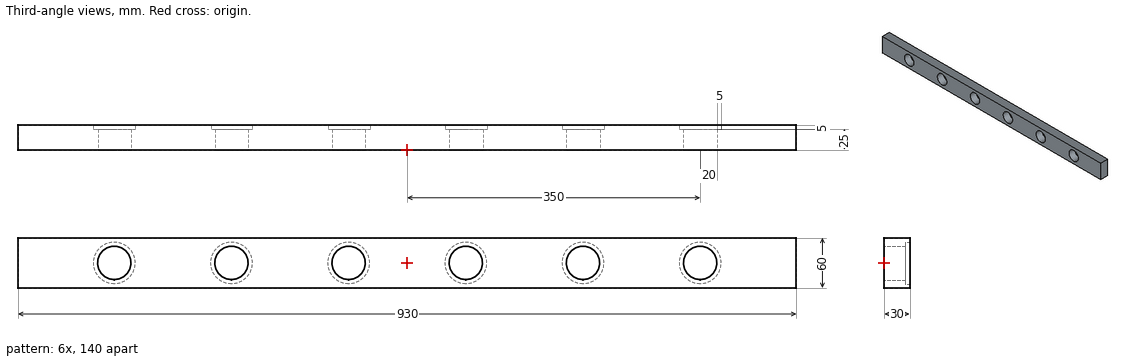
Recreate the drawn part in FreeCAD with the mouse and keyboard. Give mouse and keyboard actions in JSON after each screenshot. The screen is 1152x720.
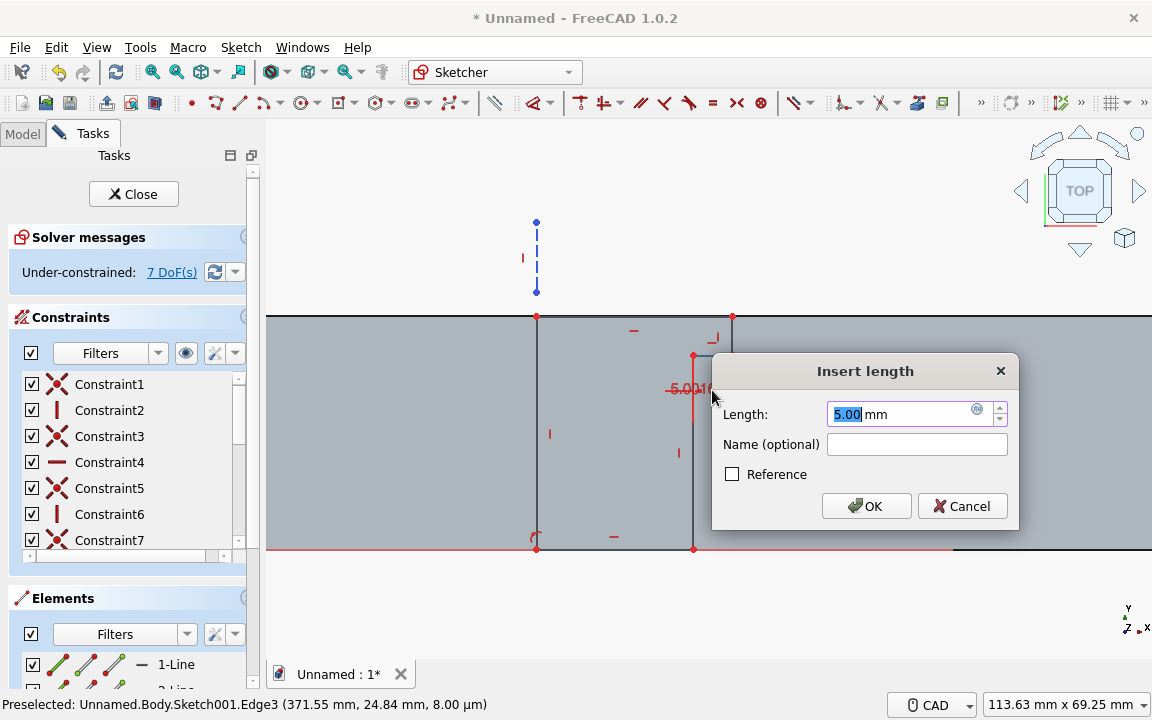
{"action": "type", "text": "5"}
{"action": "key", "text": "Return"}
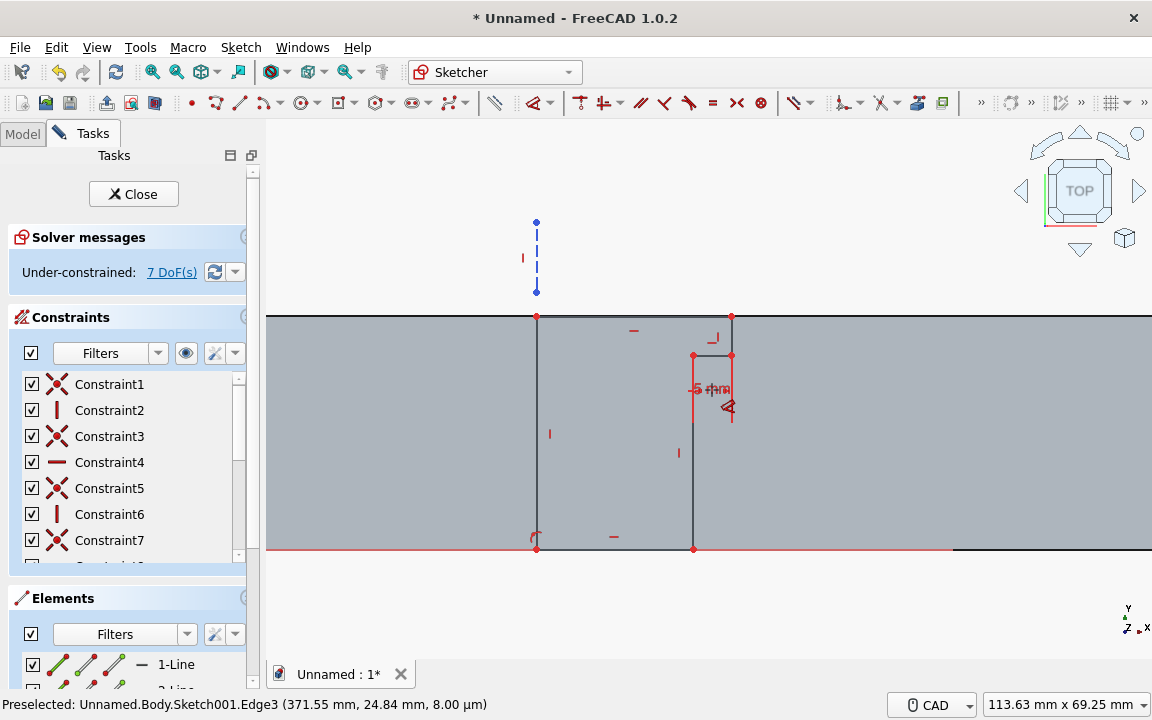
{"action": "left_click", "coordinate": [732, 344]}
{"action": "left_click", "coordinate": [766, 337]}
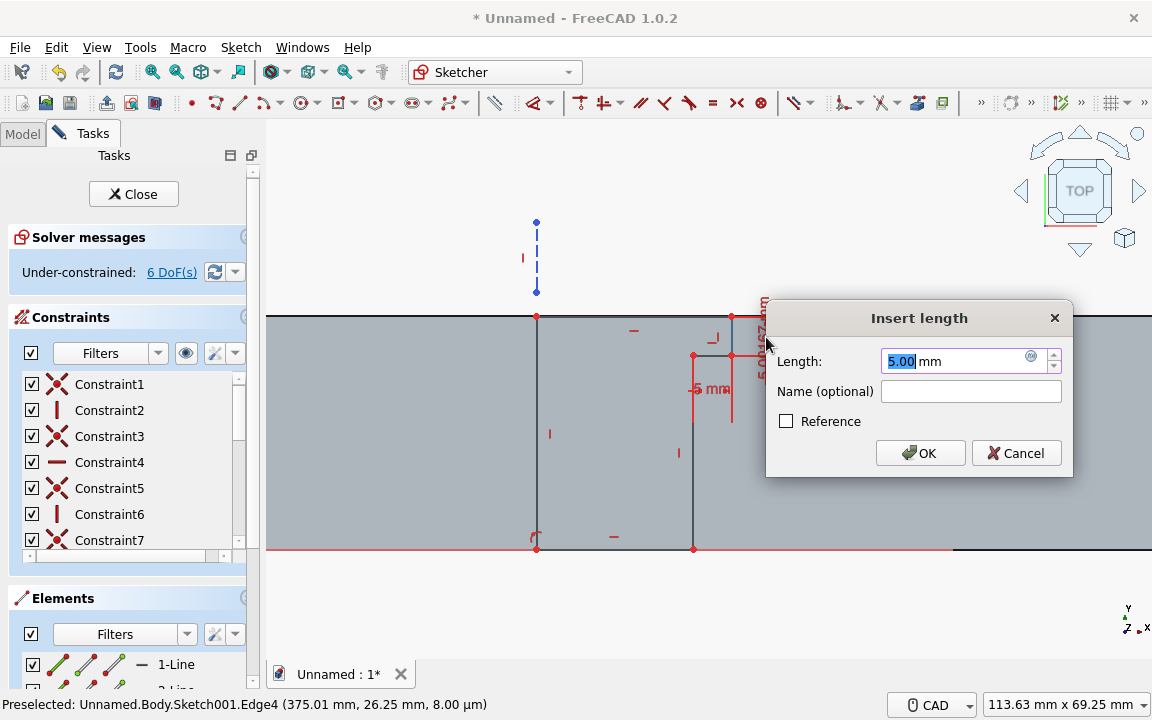
{"action": "type", "text": "5"}
{"action": "key", "text": "Return"}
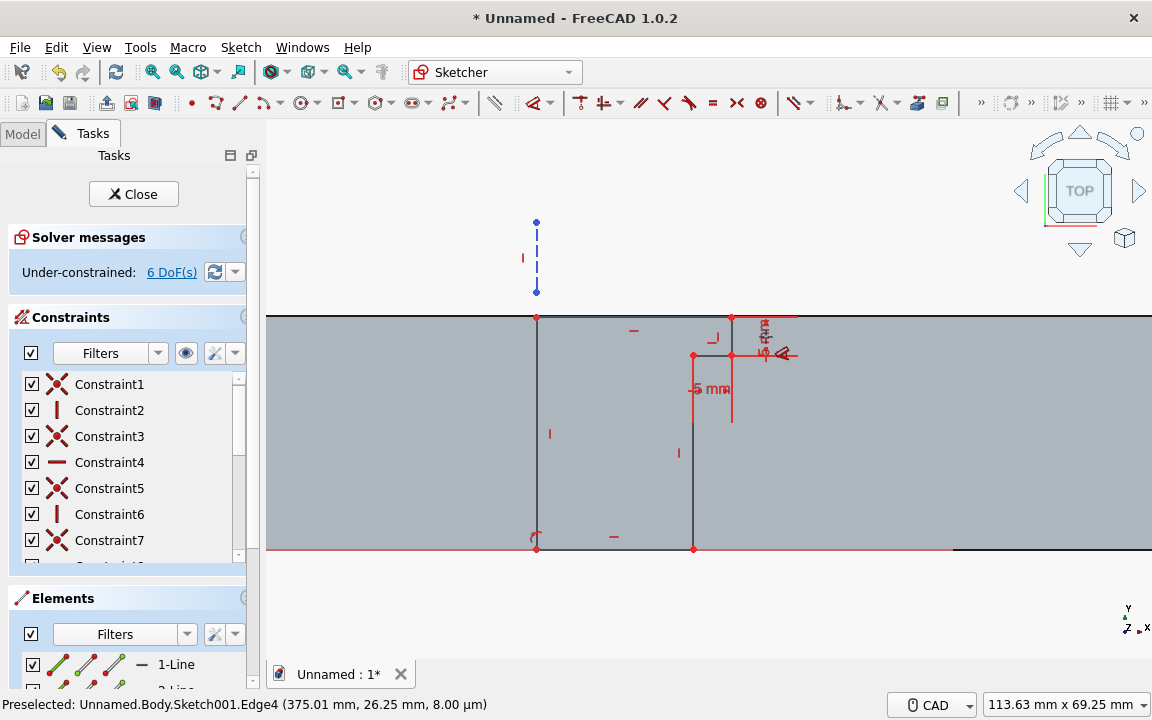
{"action": "left_click", "coordinate": [584, 550]}
{"action": "left_click", "coordinate": [615, 584]}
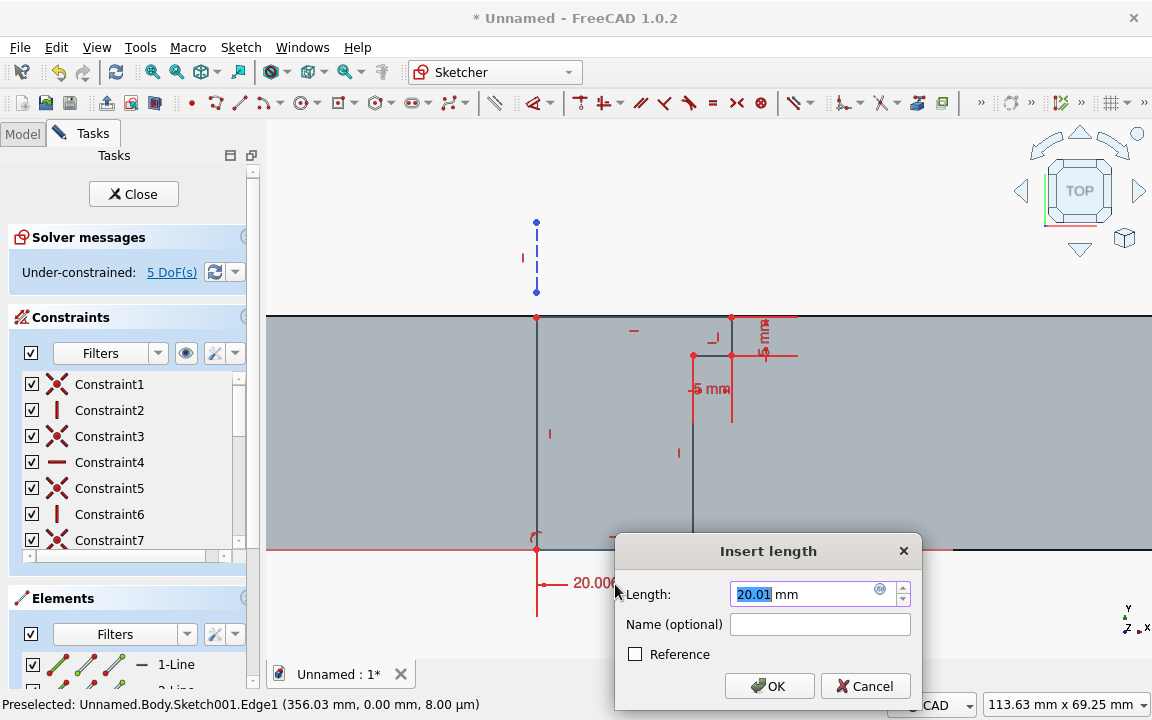
{"action": "type", "text": "20"}
{"action": "key", "text": "Return"}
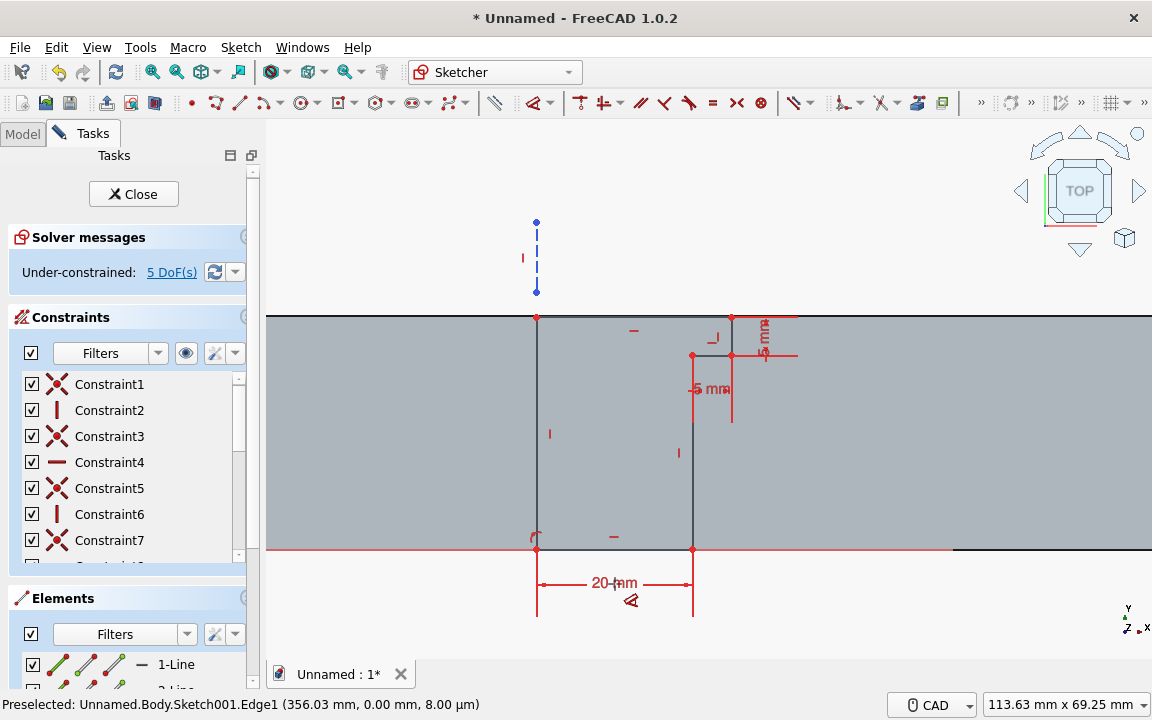
{"action": "left_click", "coordinate": [693, 492]}
{"action": "left_click", "coordinate": [727, 453]}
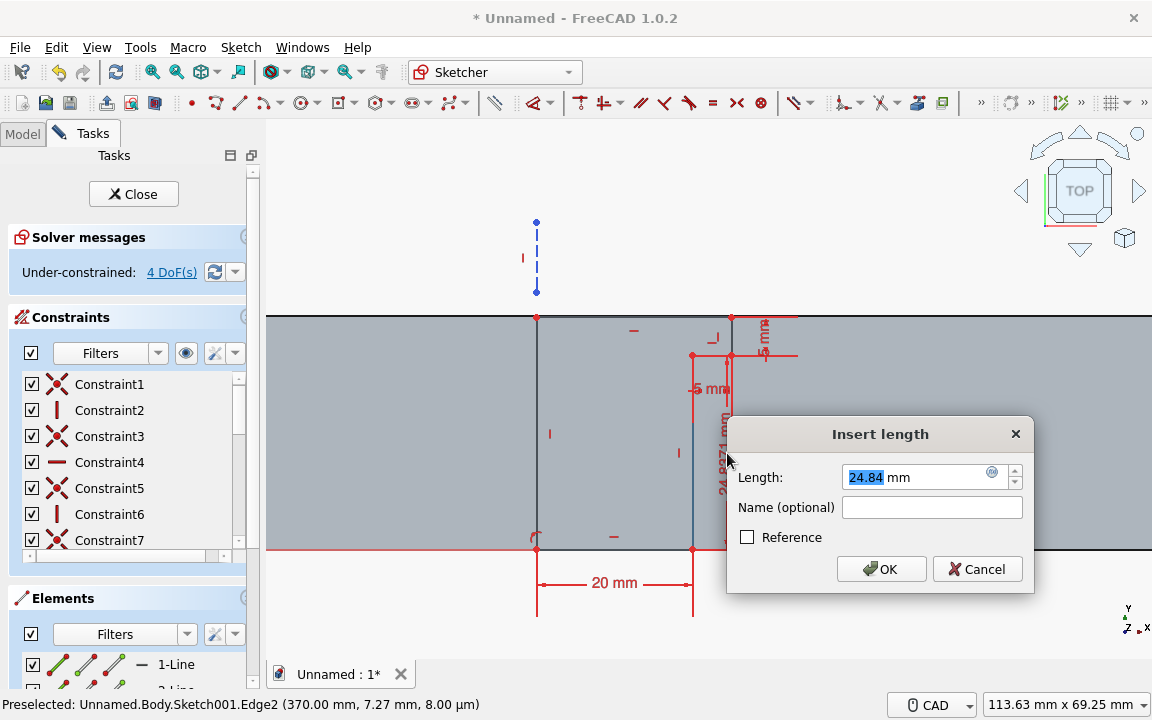
{"action": "type", "text": "25"}
{"action": "key", "text": "Return"}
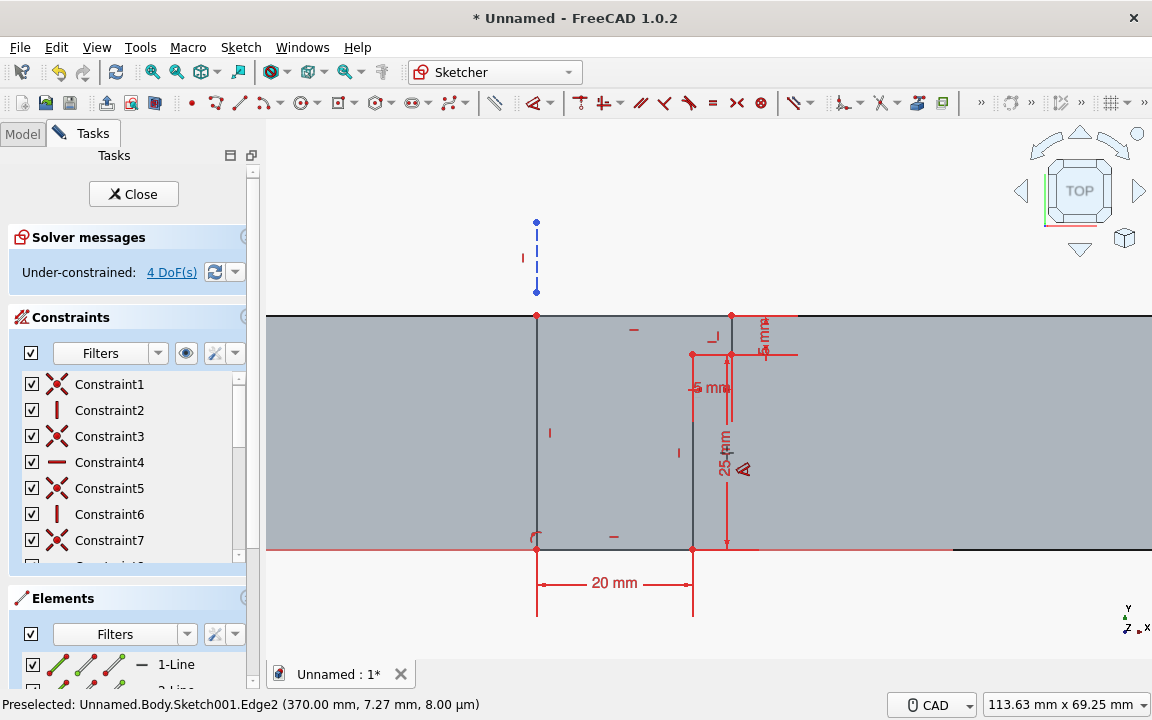
{"action": "left_click", "coordinate": [537, 550]}
{"action": "left_click", "coordinate": [415, 584]}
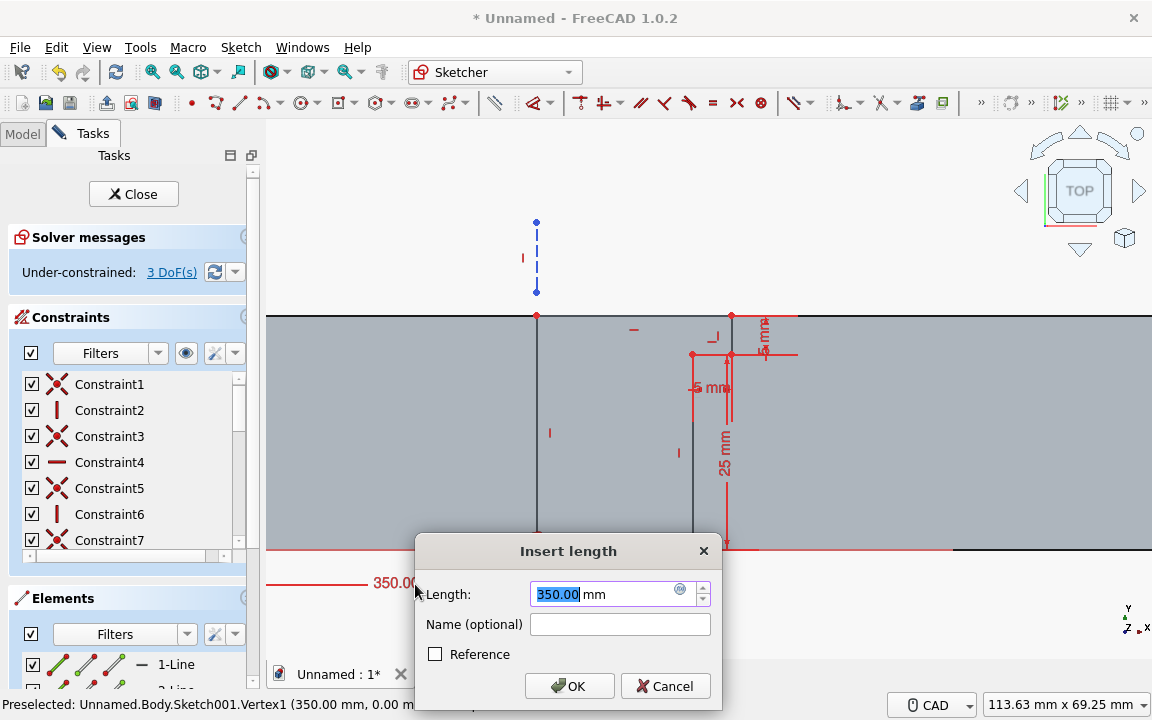
{"action": "type", "text": "350"}
{"action": "key", "text": "Return"}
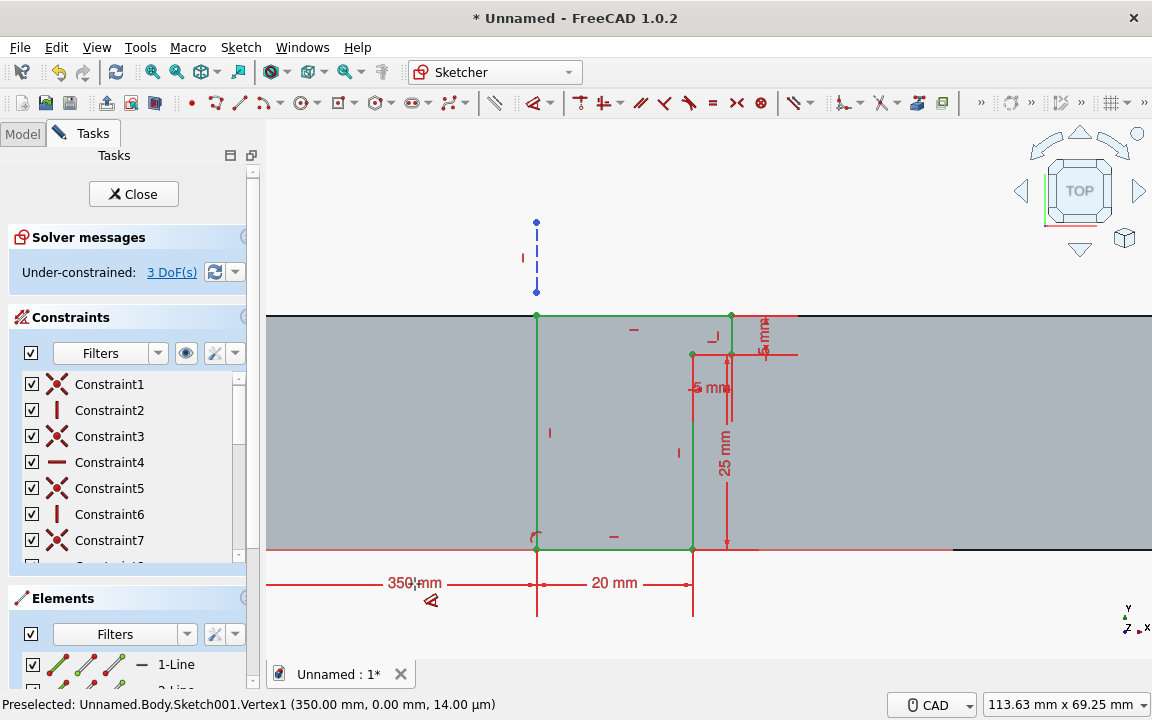
{"action": "left_click", "coordinate": [537, 293]}
{"action": "left_click", "coordinate": [330, 584]}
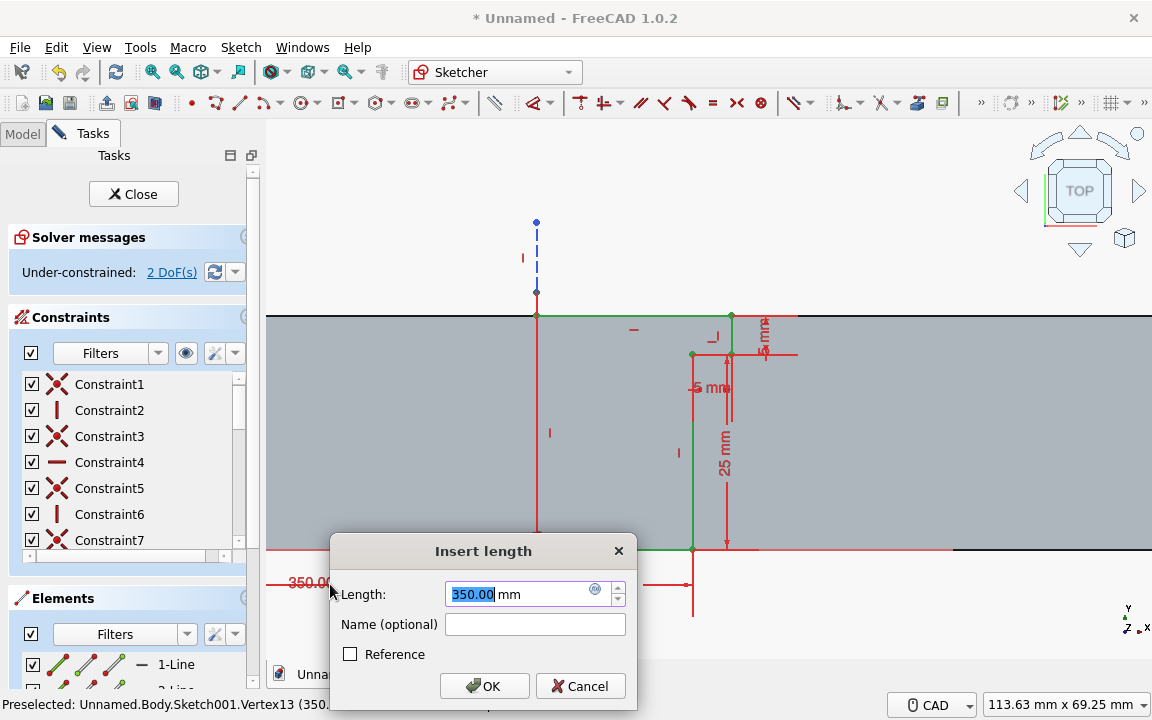
{"action": "type", "text": "350"}
{"action": "key", "text": "Return"}
{"action": "key", "text": "Escape"}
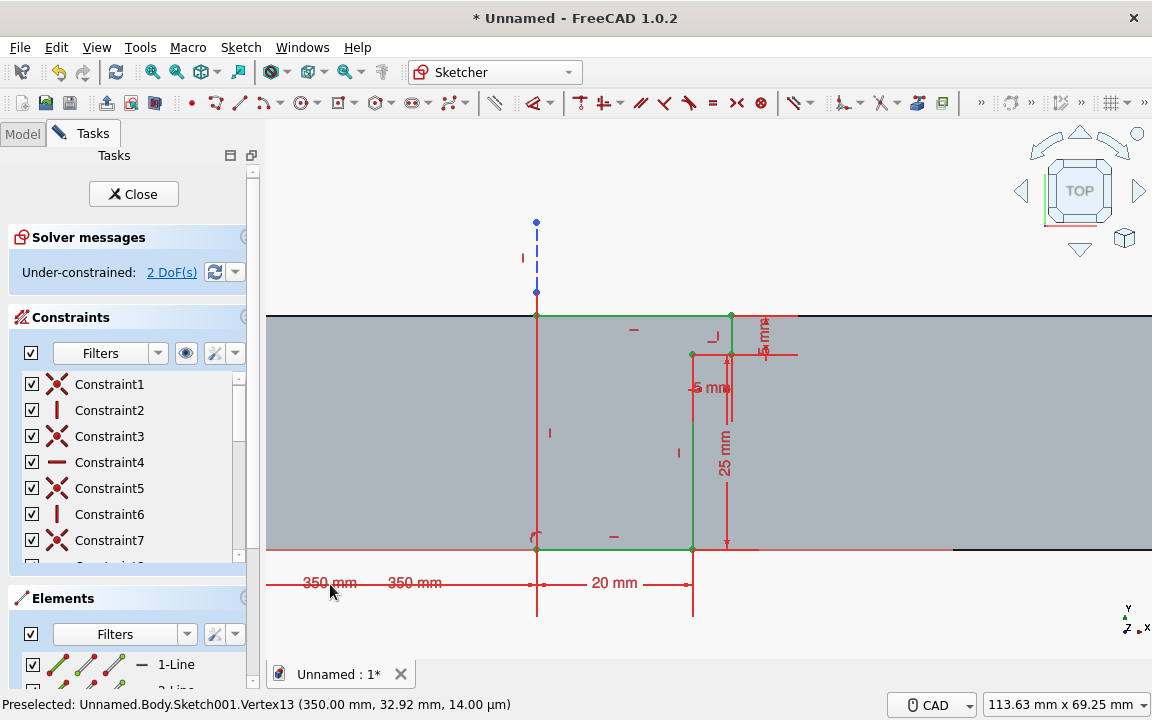
{"action": "left_click", "coordinate": [134, 194]}